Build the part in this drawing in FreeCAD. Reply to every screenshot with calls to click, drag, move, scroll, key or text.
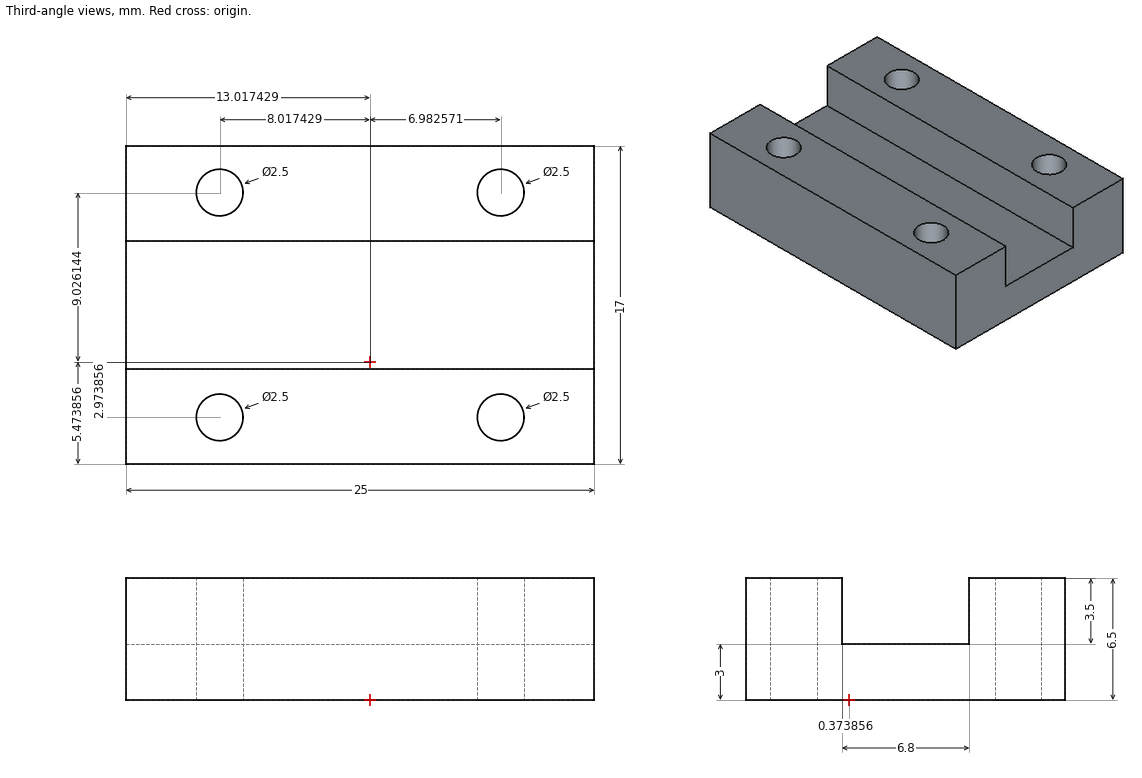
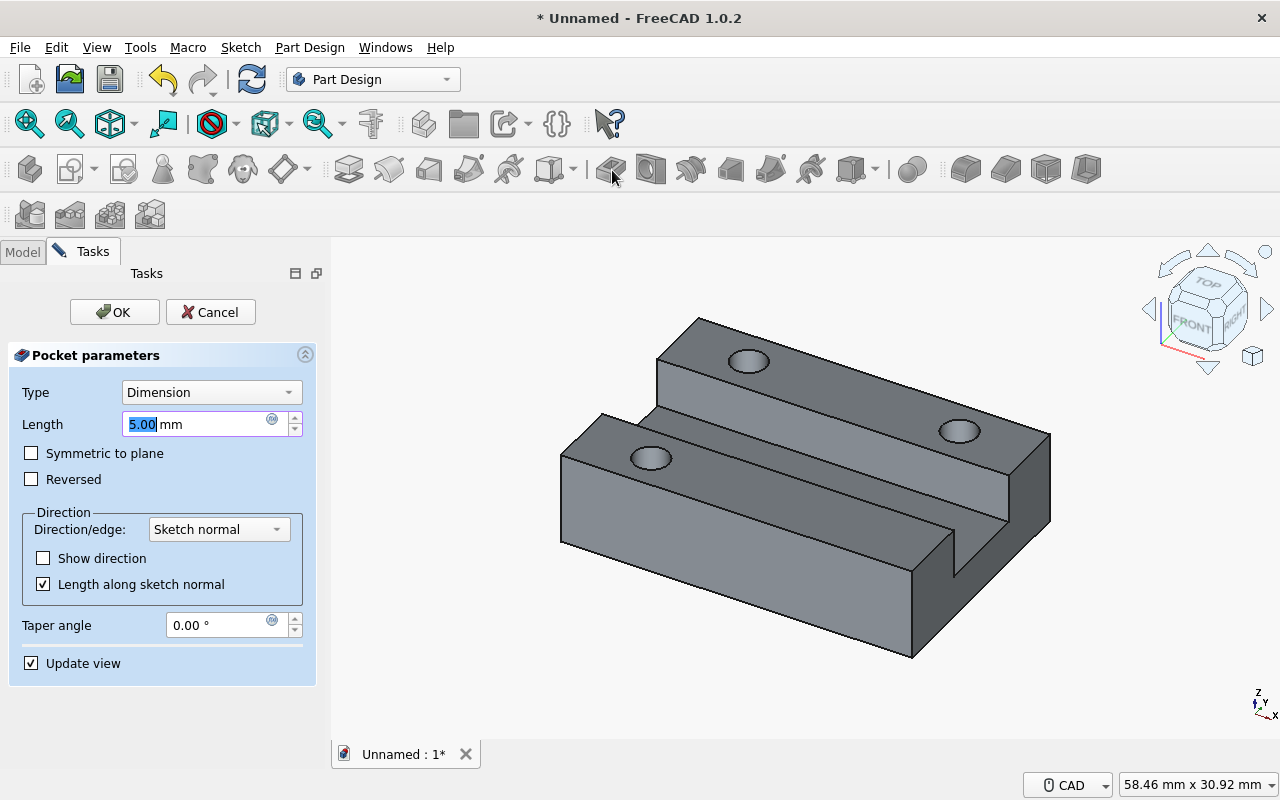
click(212, 392)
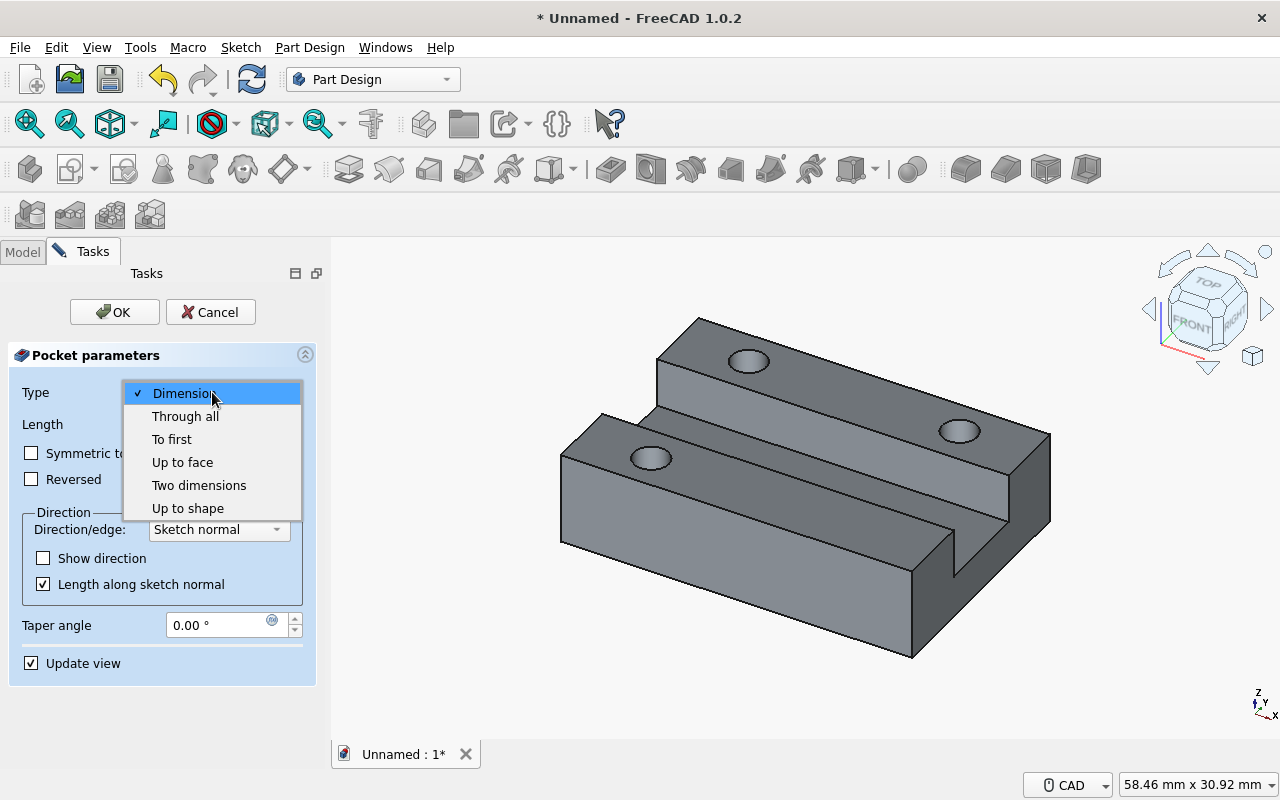
click(212, 440)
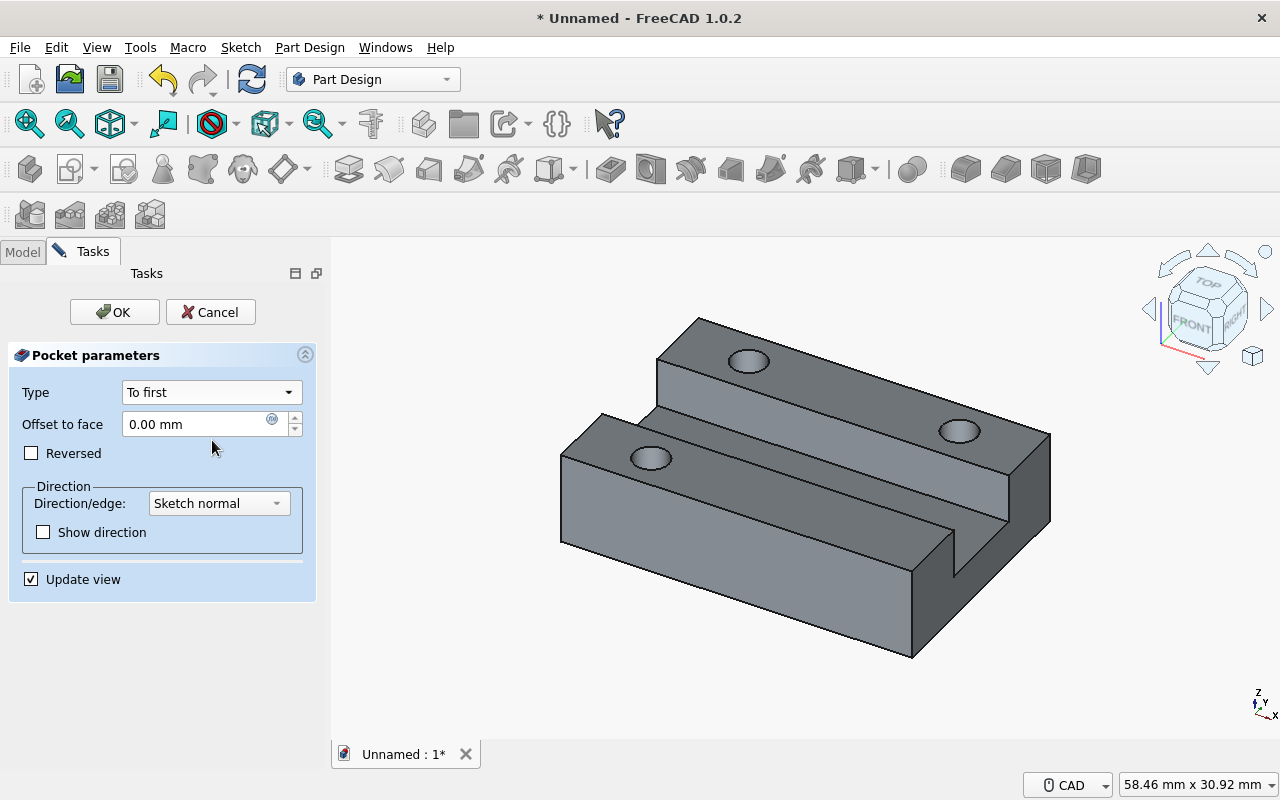
click(115, 312)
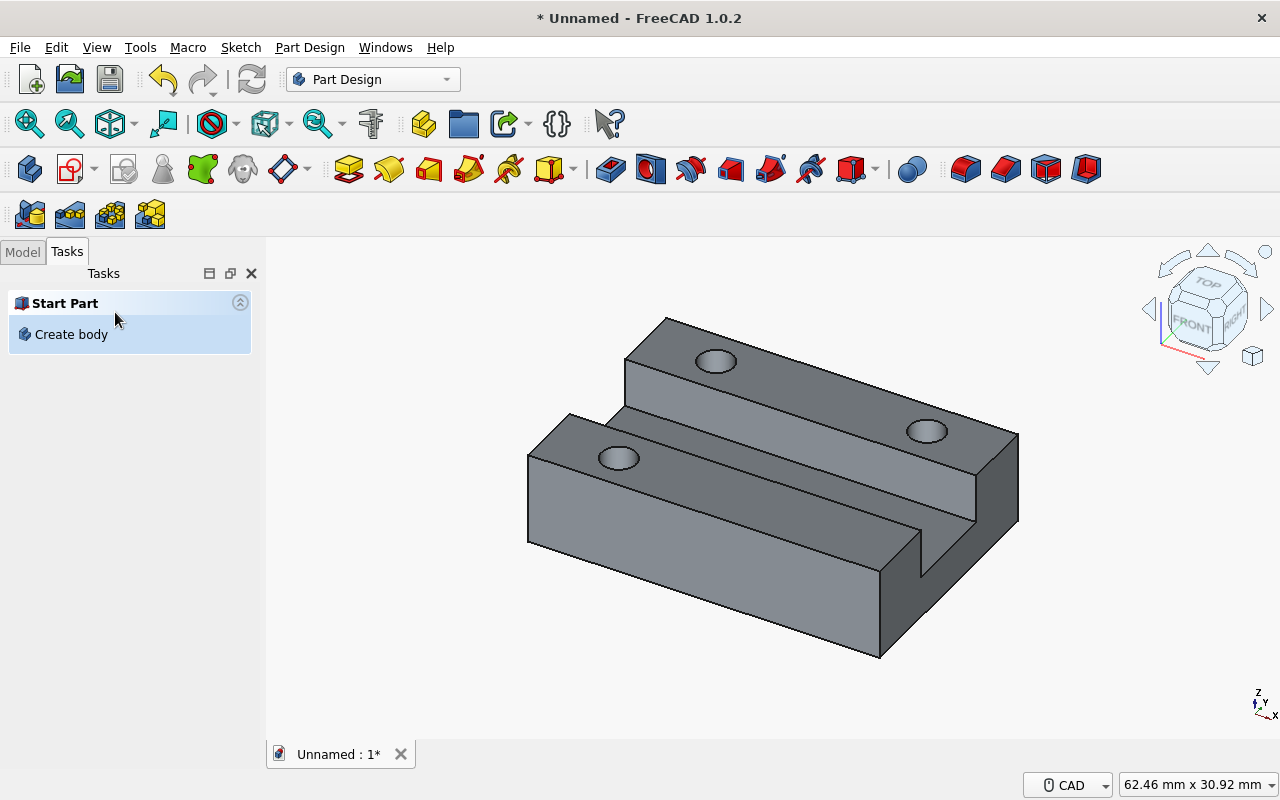
click(825, 525)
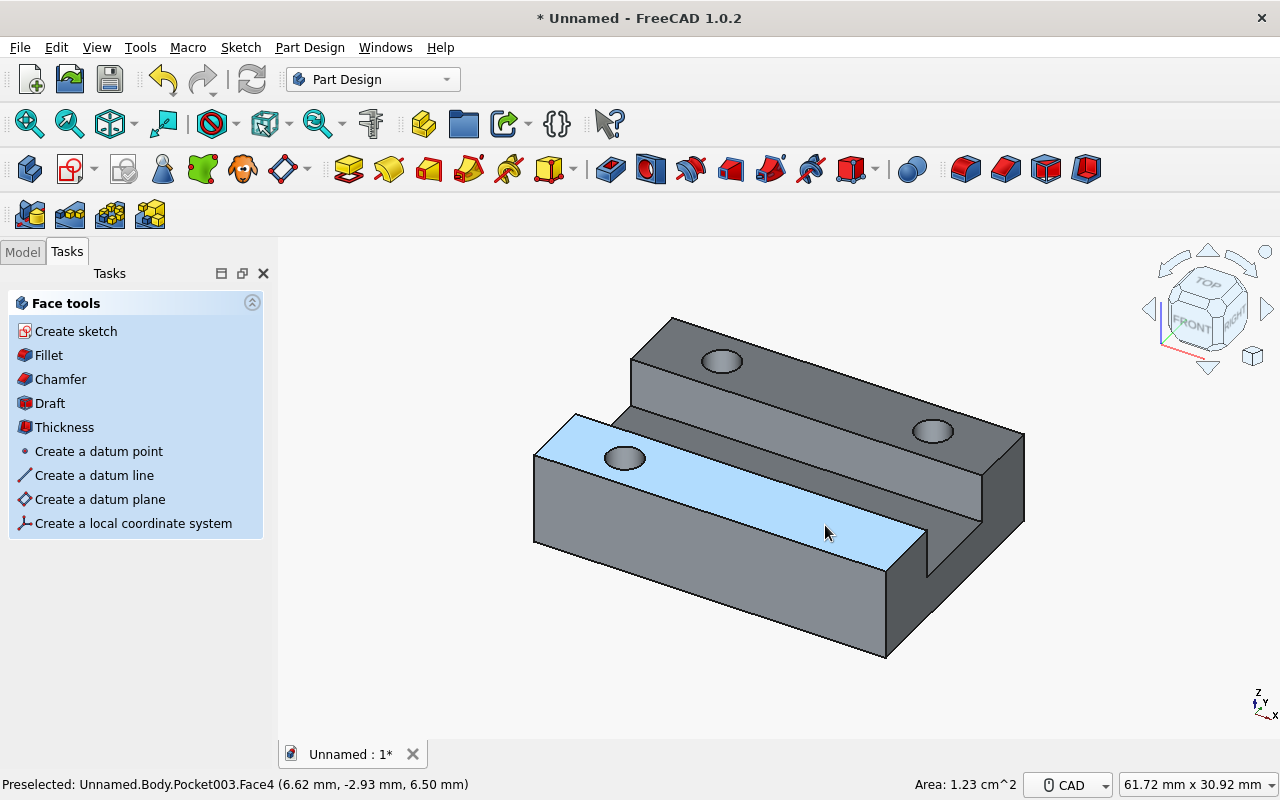
click(70, 170)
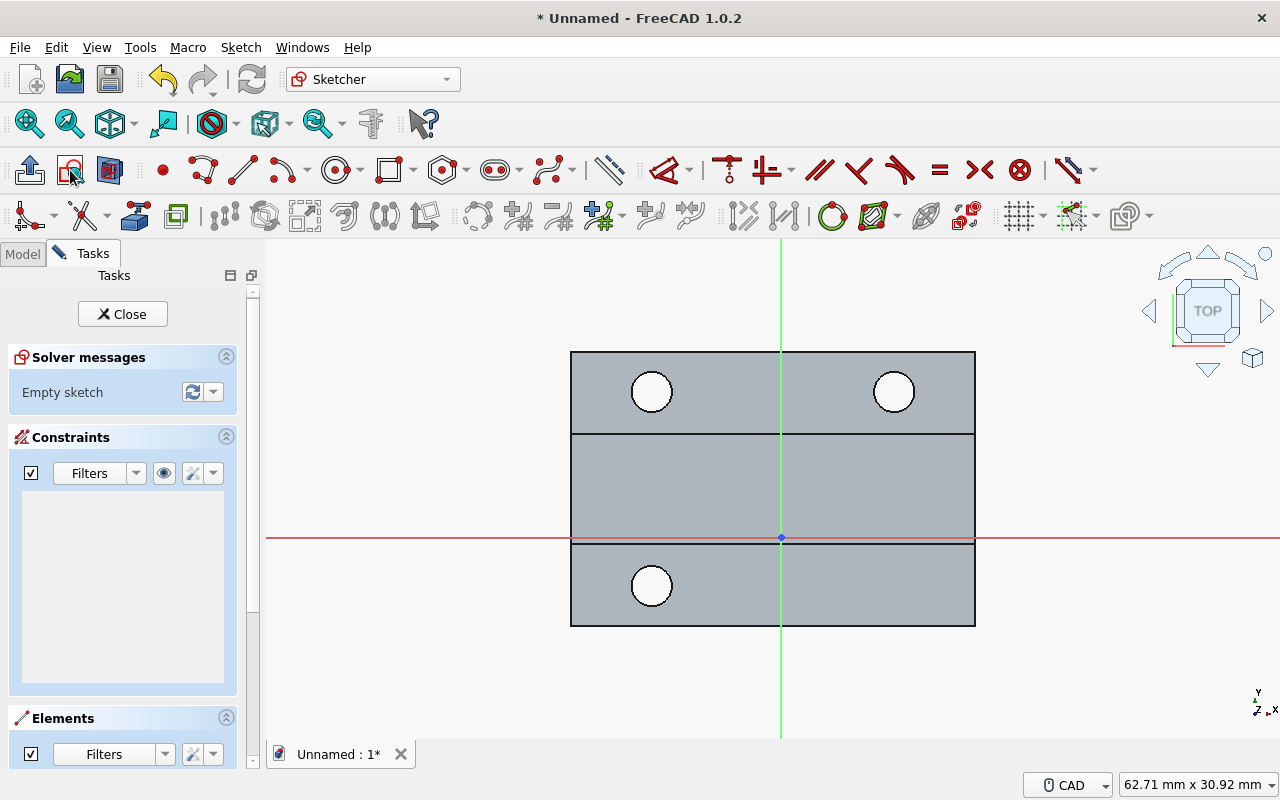
scroll(924, 601, up, 10)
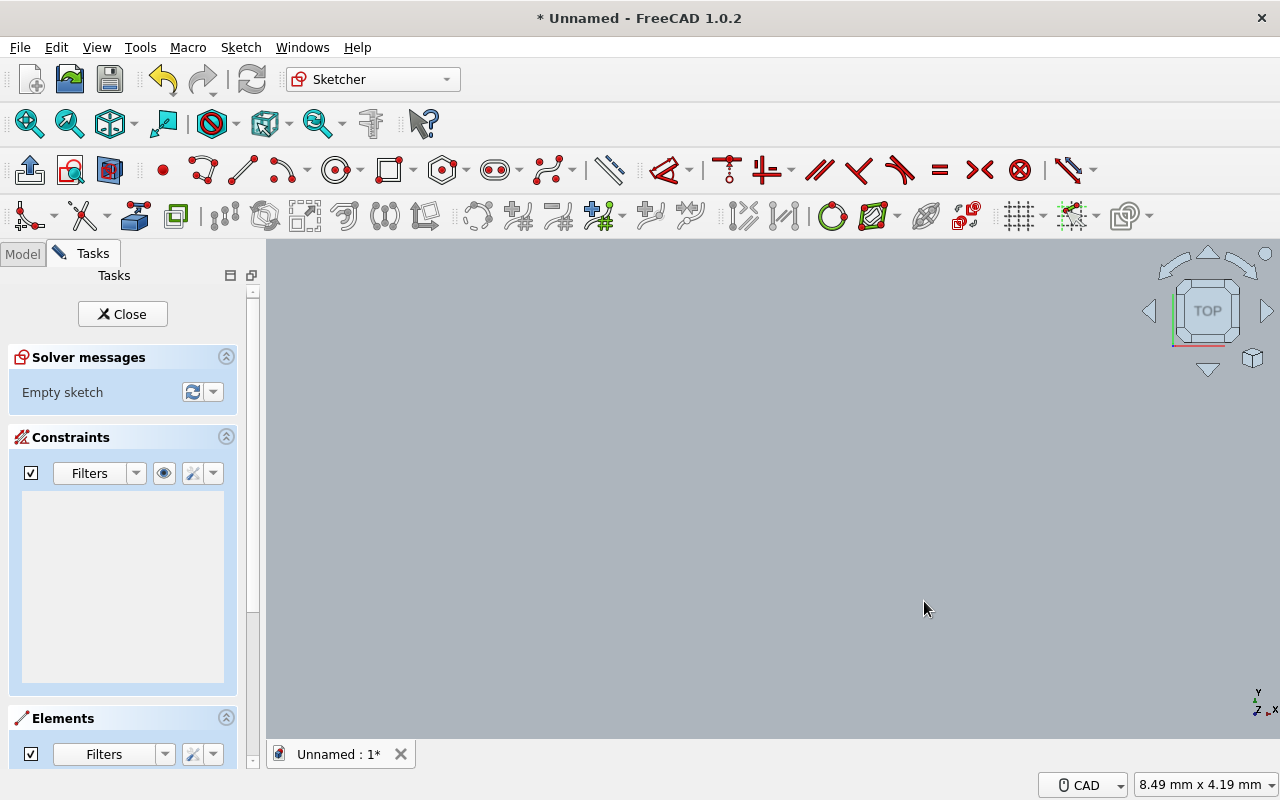
click(336, 170)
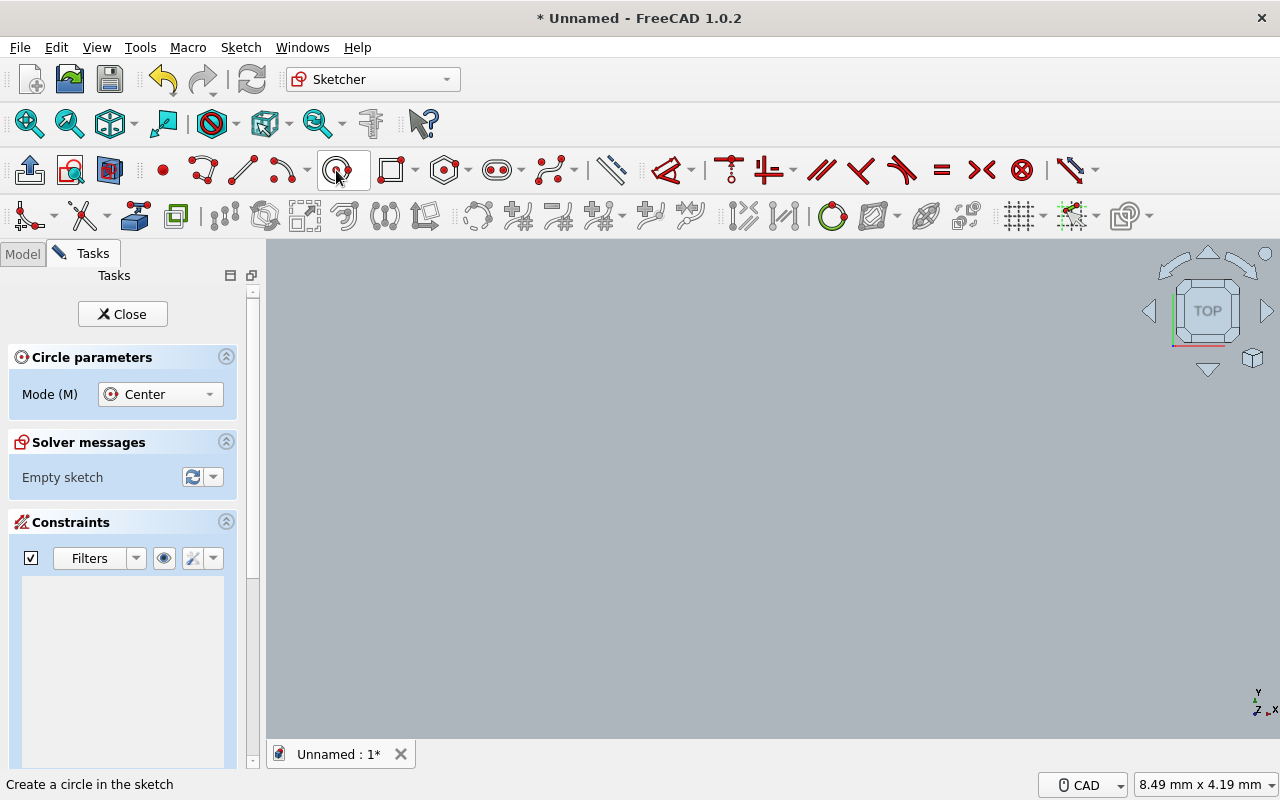
click(700, 486)
move(806, 380)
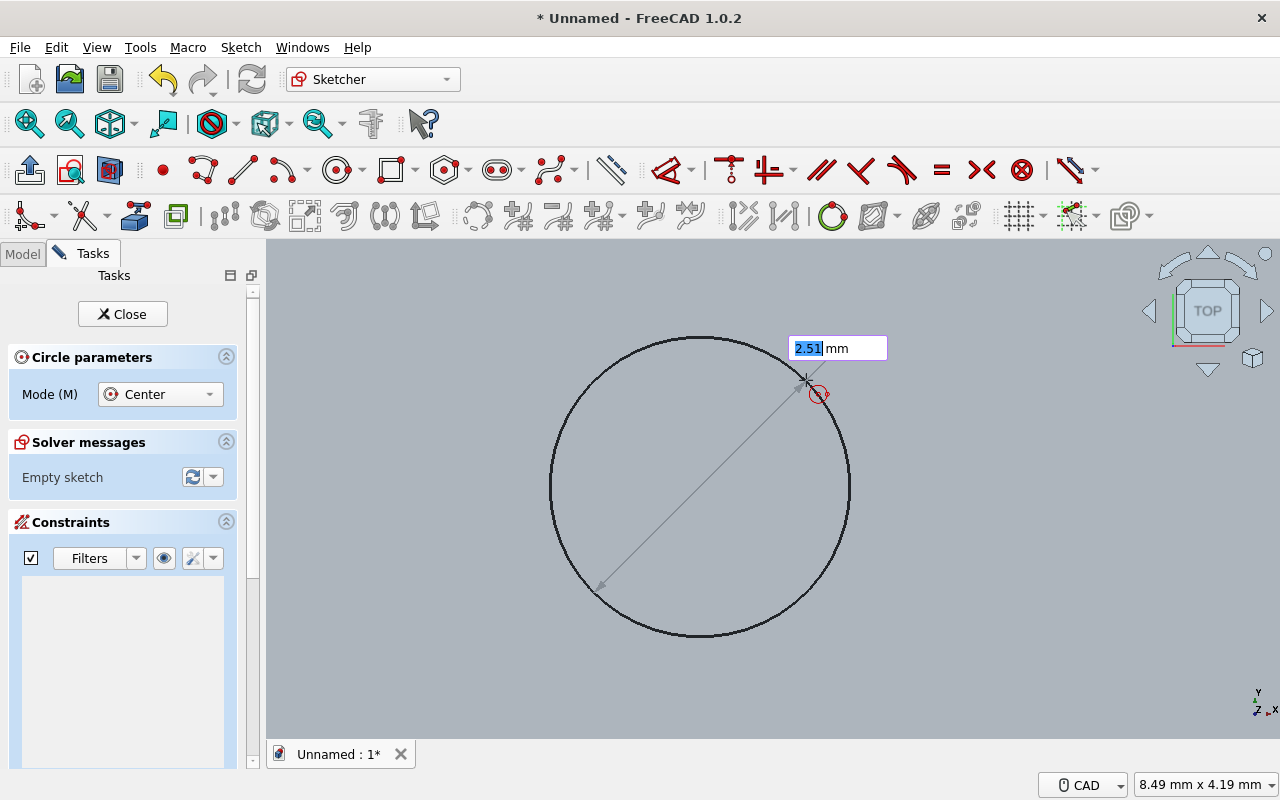
text(2.5)
key(Return)
key(Escape)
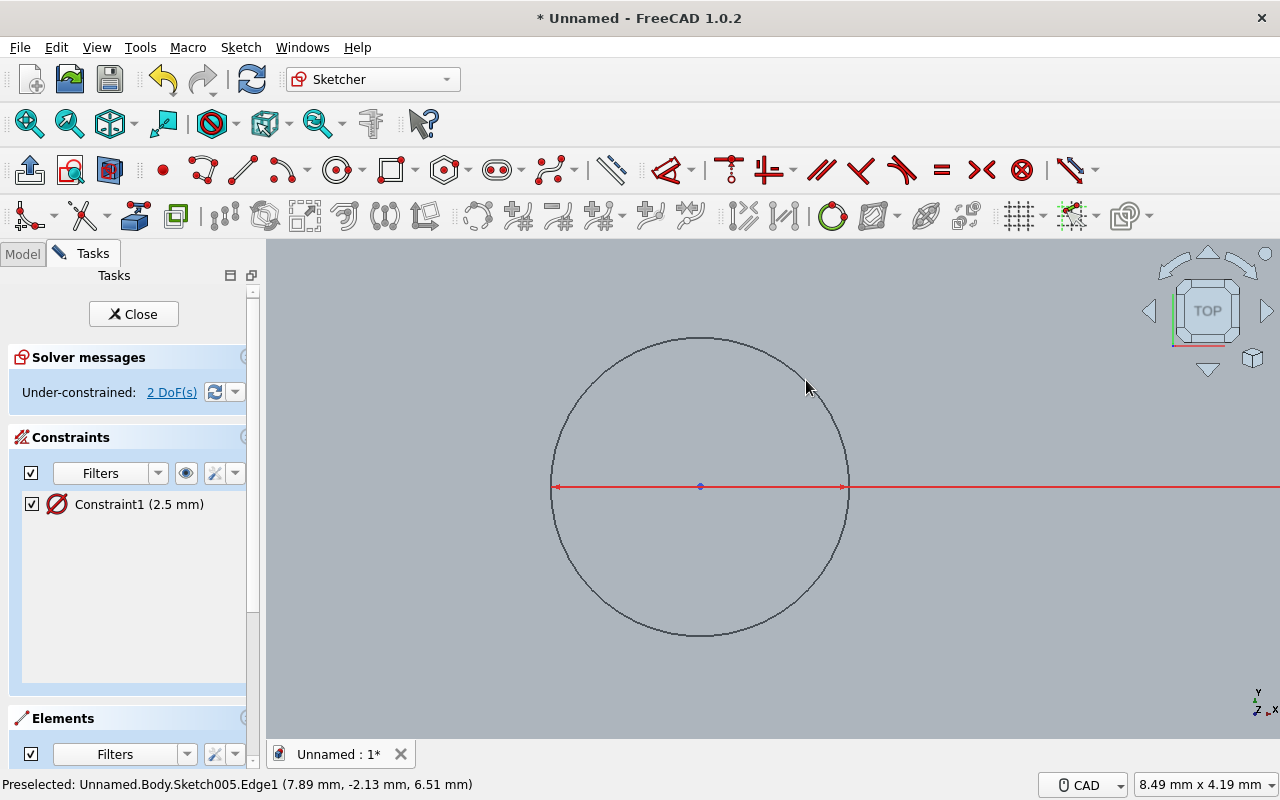
key(d)